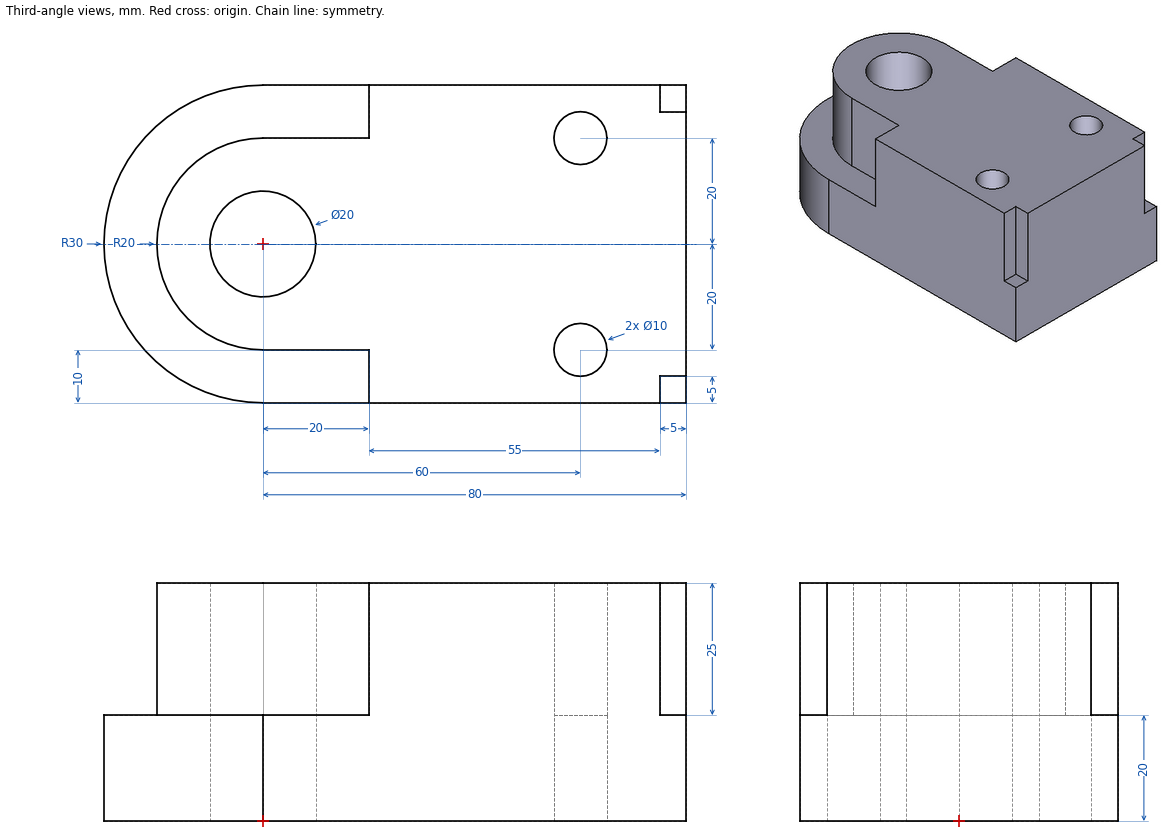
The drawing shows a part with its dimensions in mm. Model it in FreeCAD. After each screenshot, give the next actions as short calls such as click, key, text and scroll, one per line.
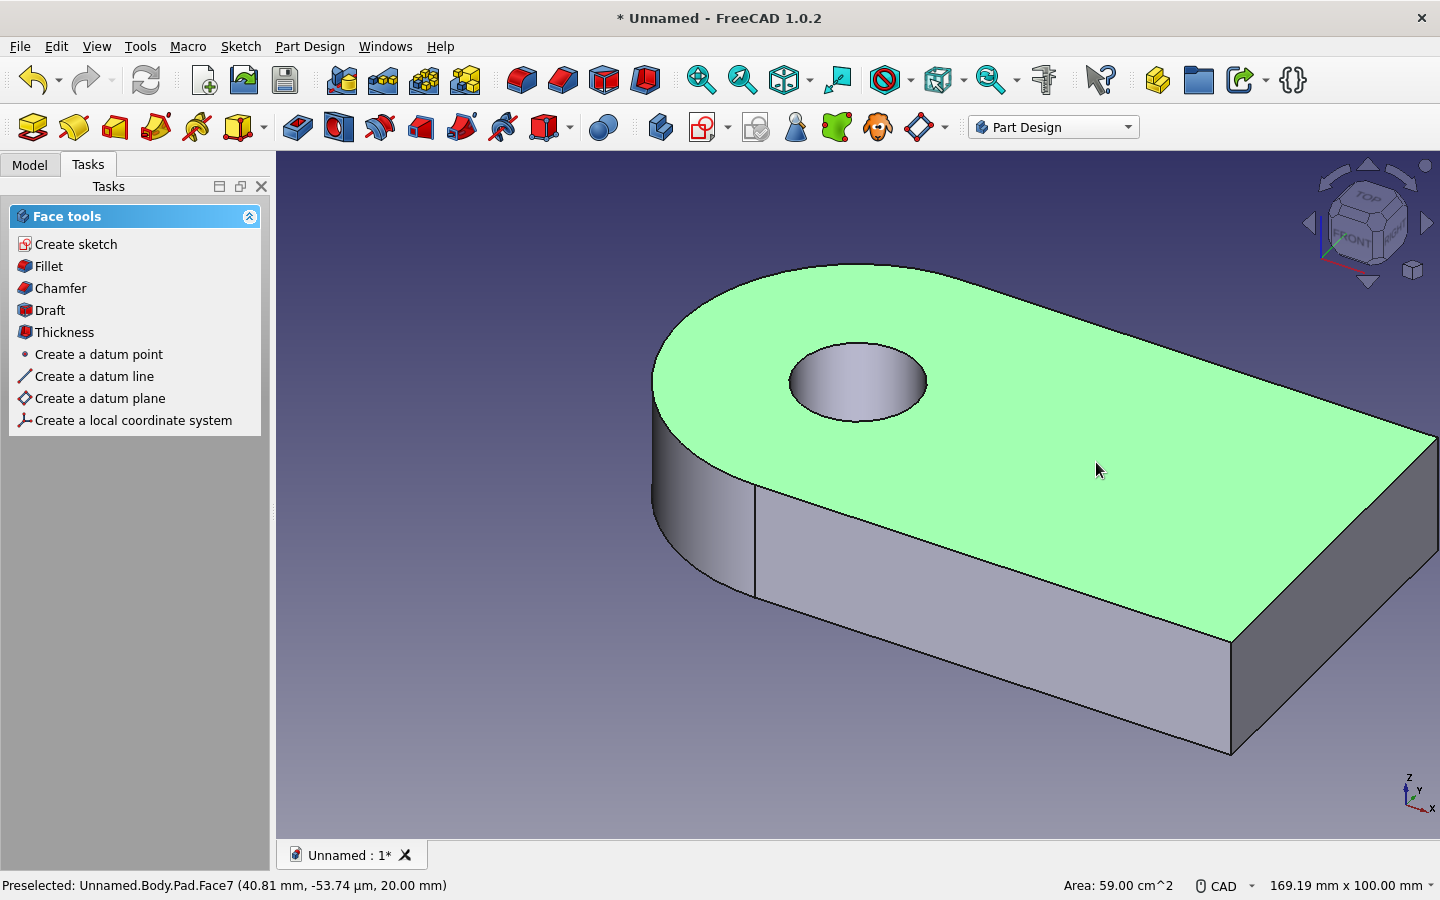
click(702, 128)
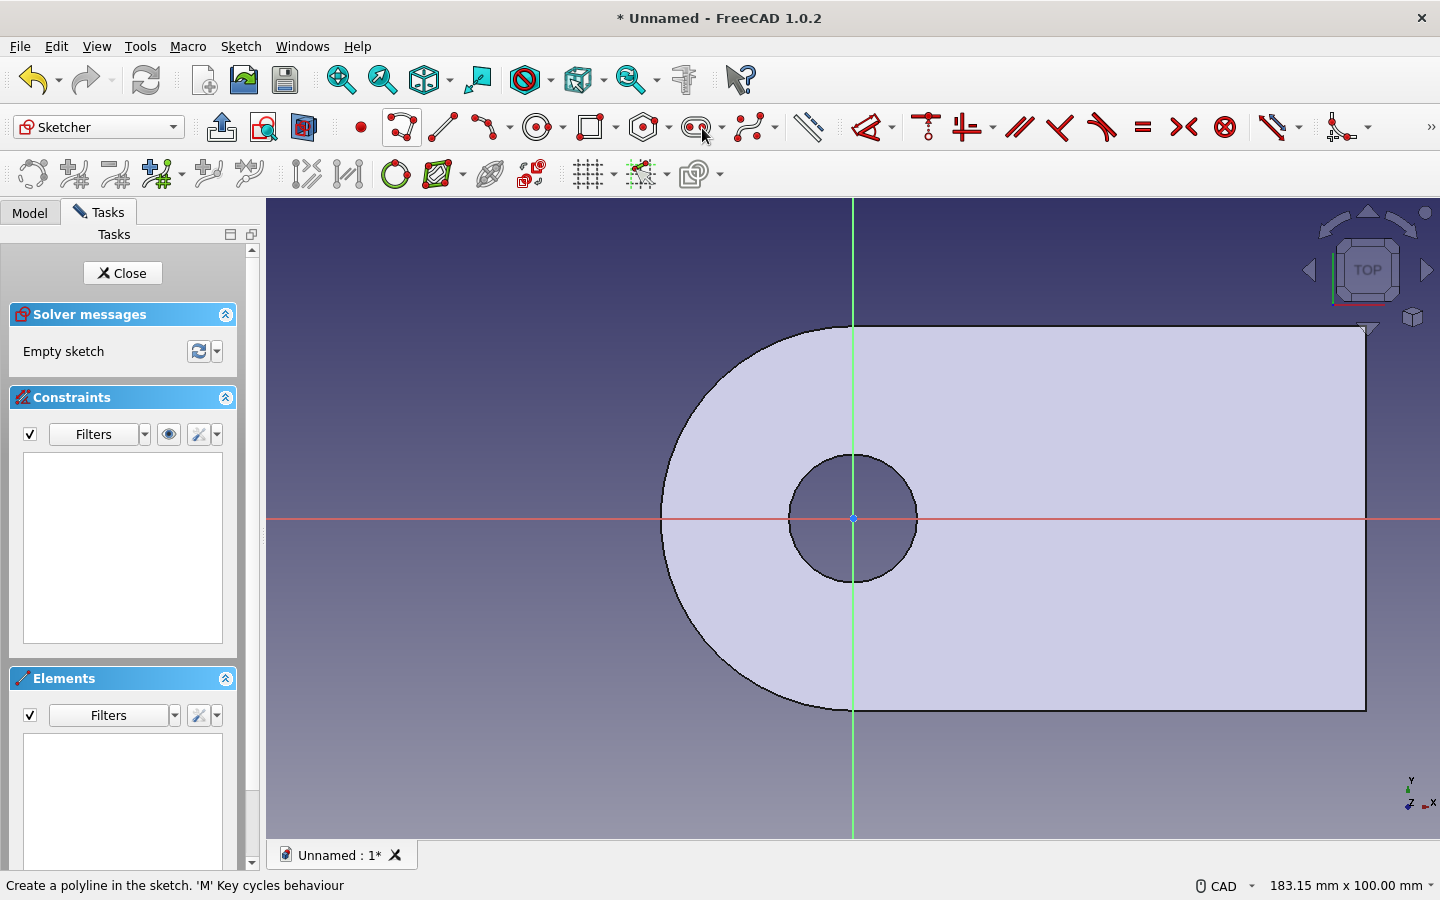
scroll(294, 519, down, 1)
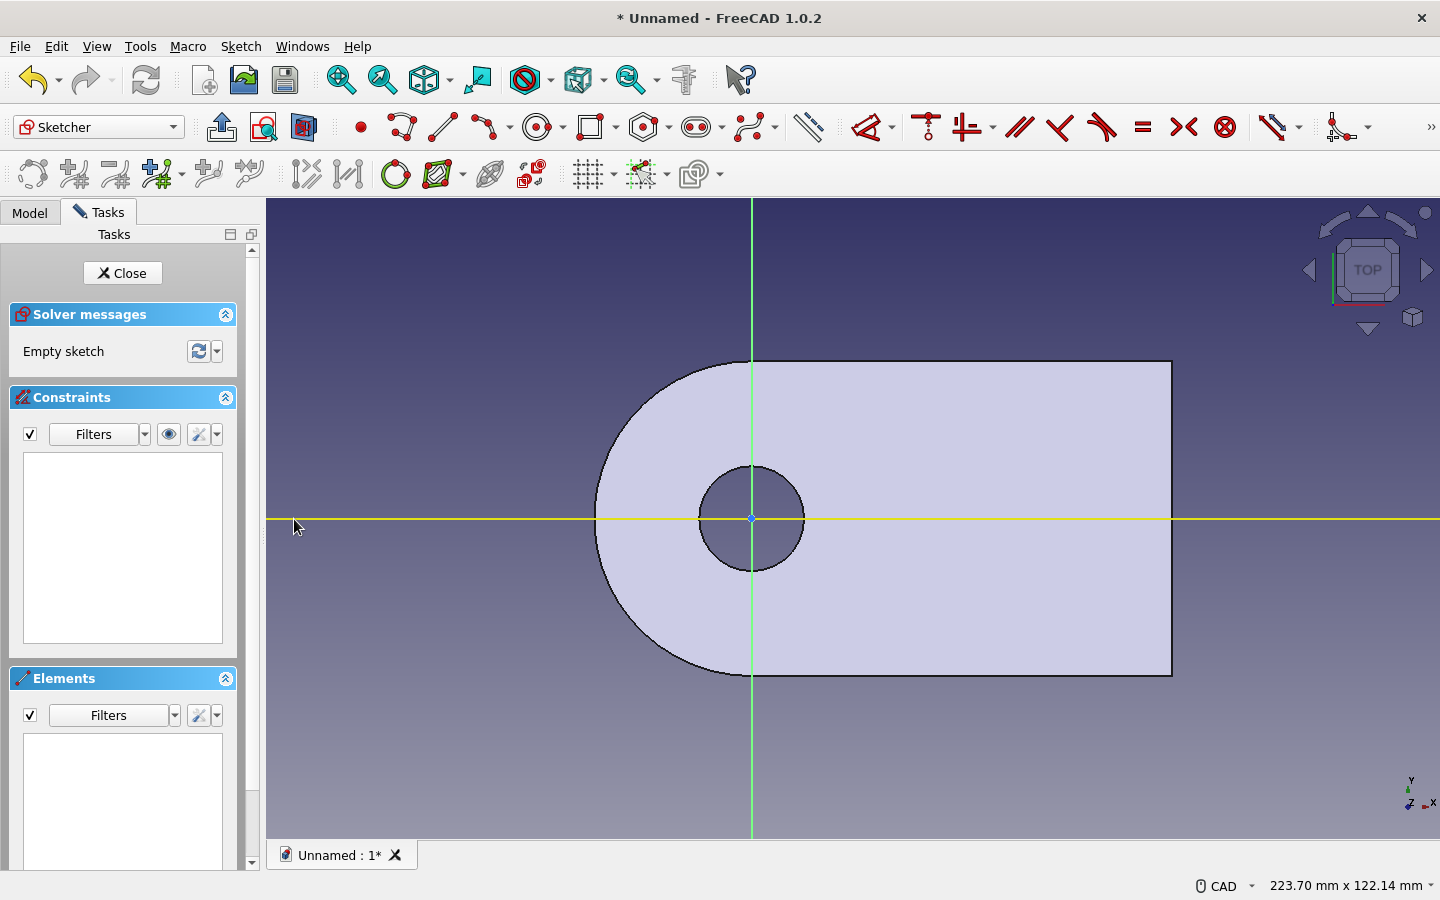
click(402, 128)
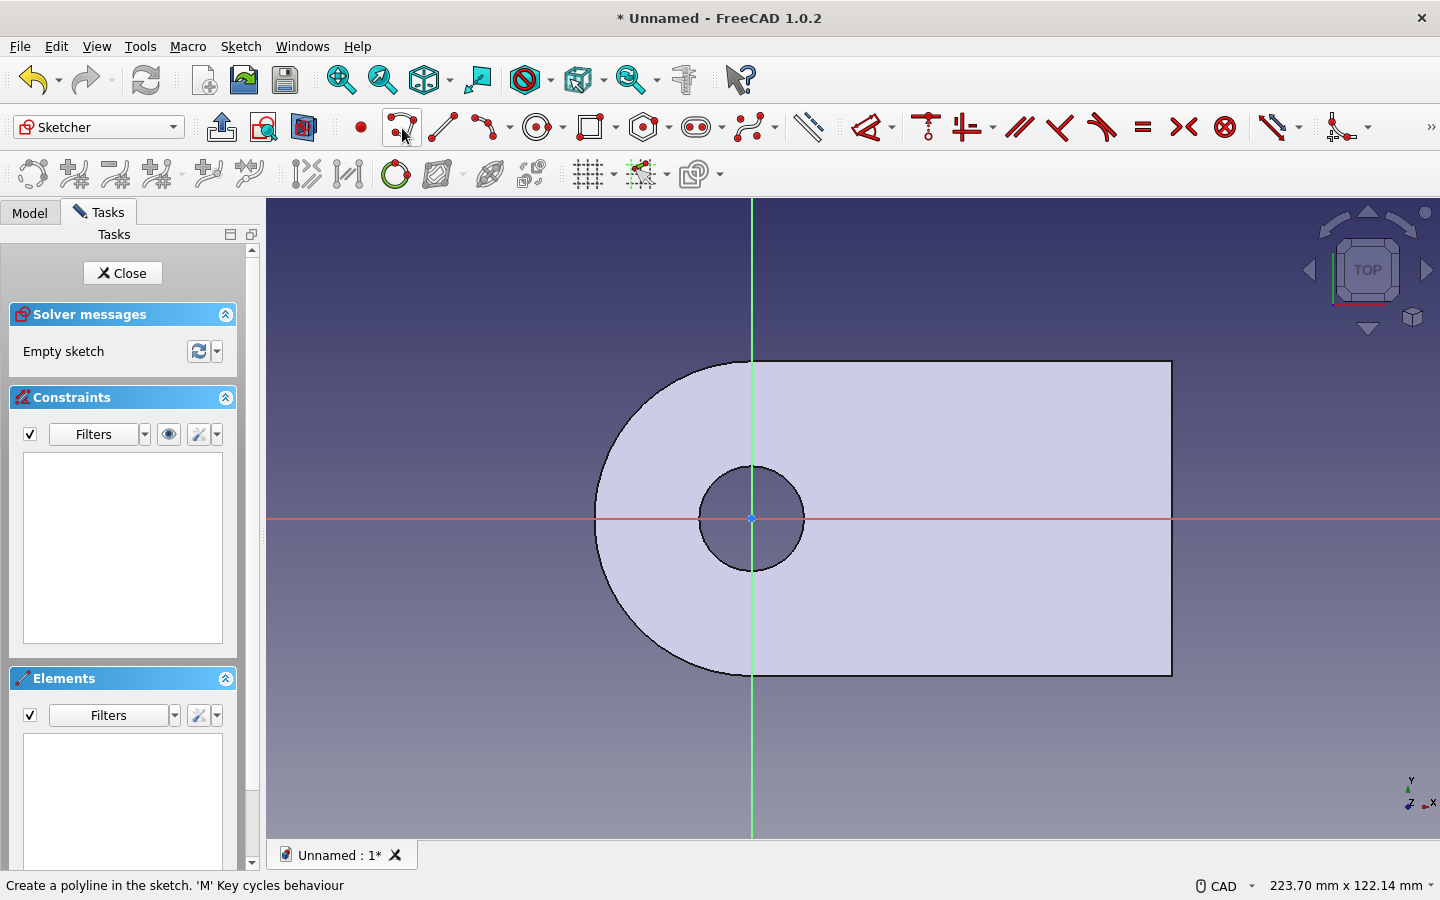
click(752, 624)
click(857, 624)
click(857, 676)
click(1145, 676)
click(1145, 650)
click(1172, 650)
click(1172, 387)
click(1145, 387)
click(1145, 361)
click(857, 361)
click(857, 414)
click(752, 414)
right_click(752, 414)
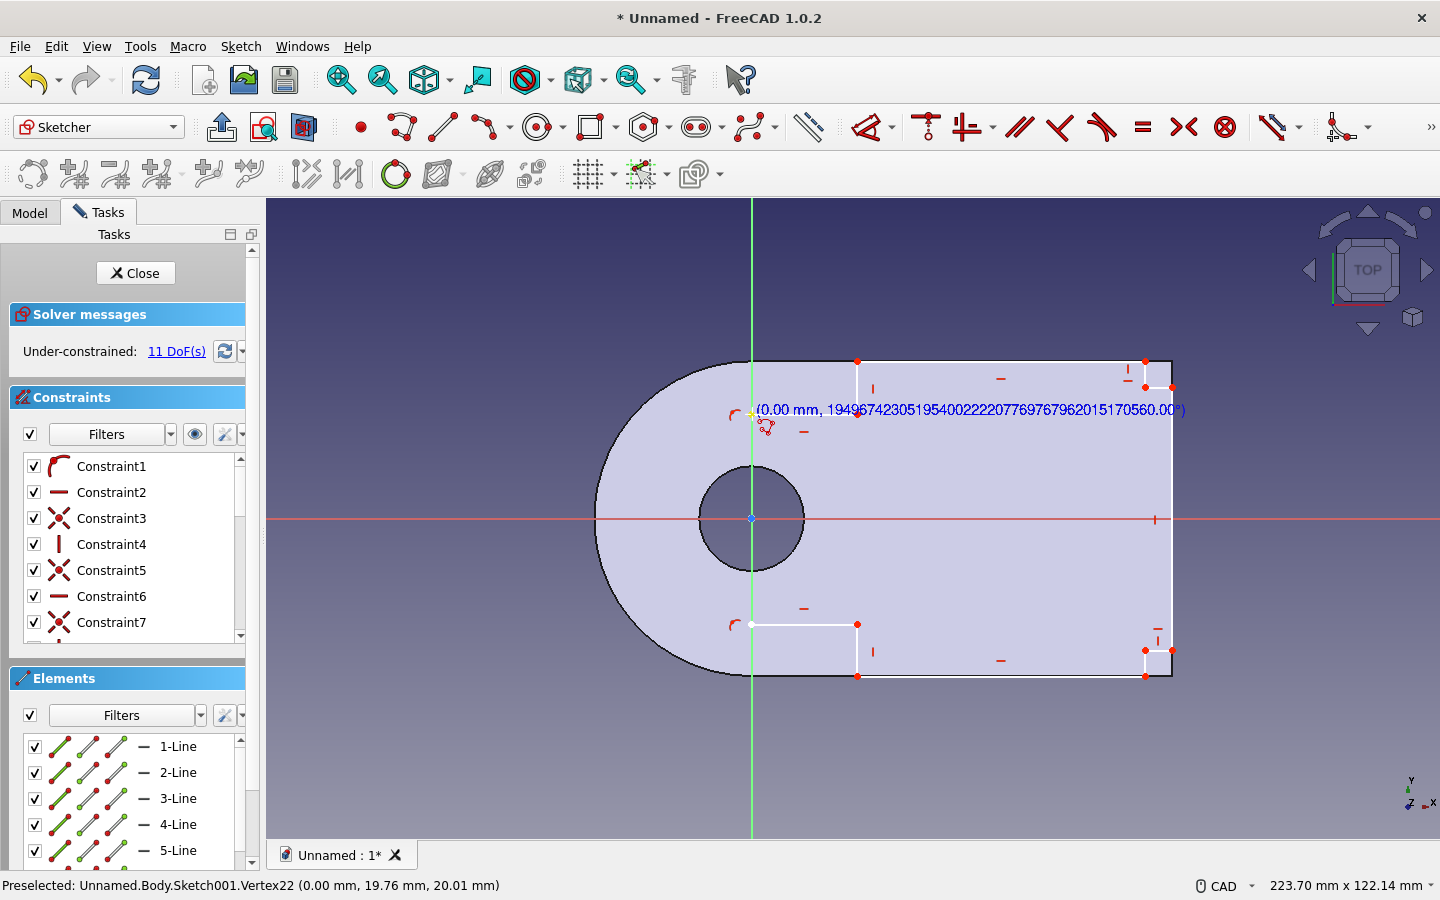
key(g)
key(3)
key(a)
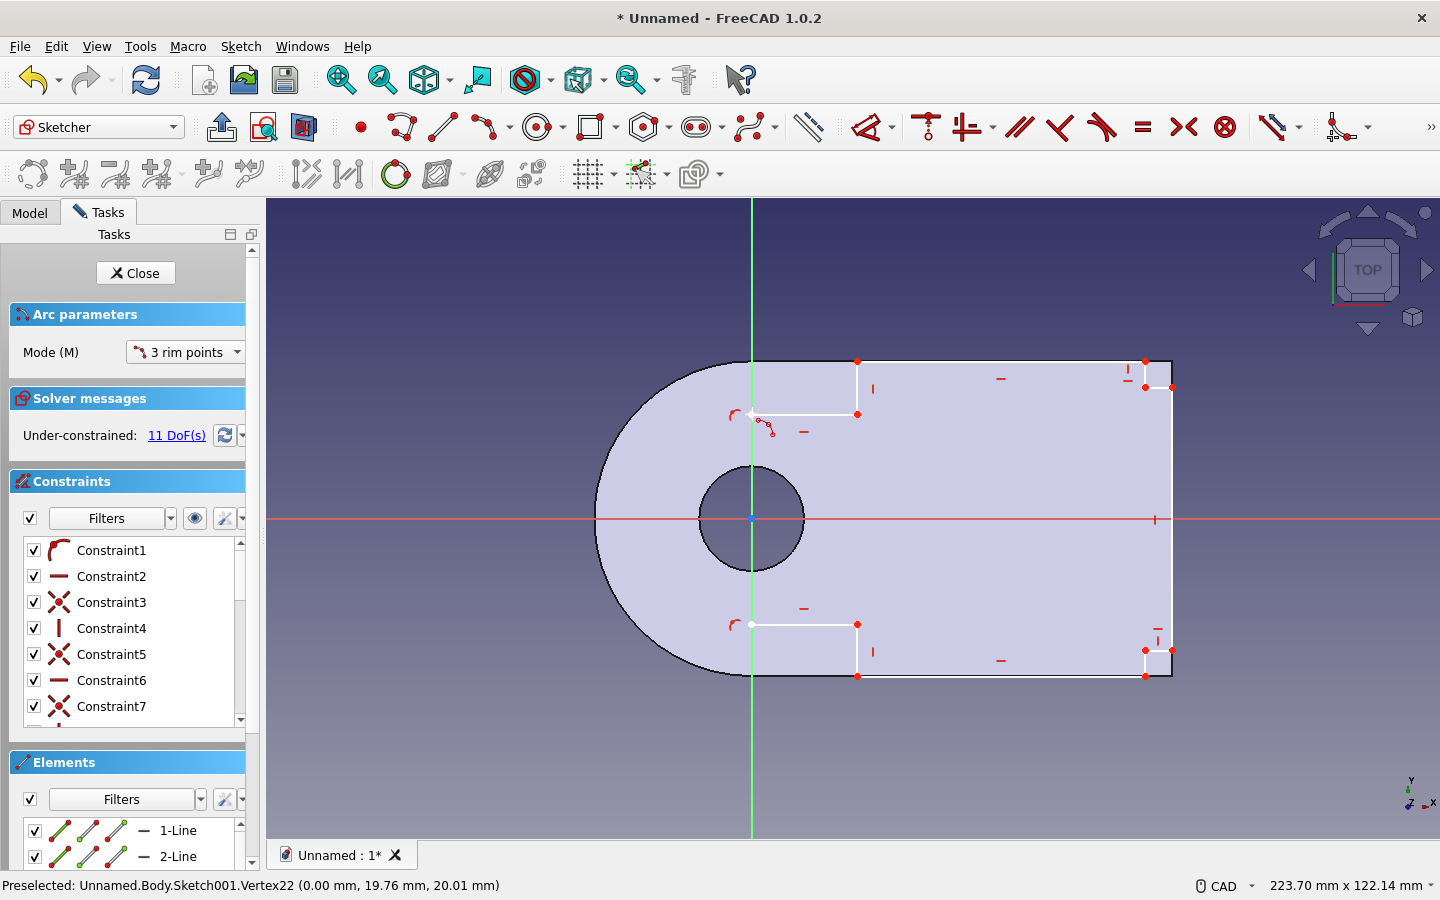
click(752, 415)
click(752, 625)
click(652, 486)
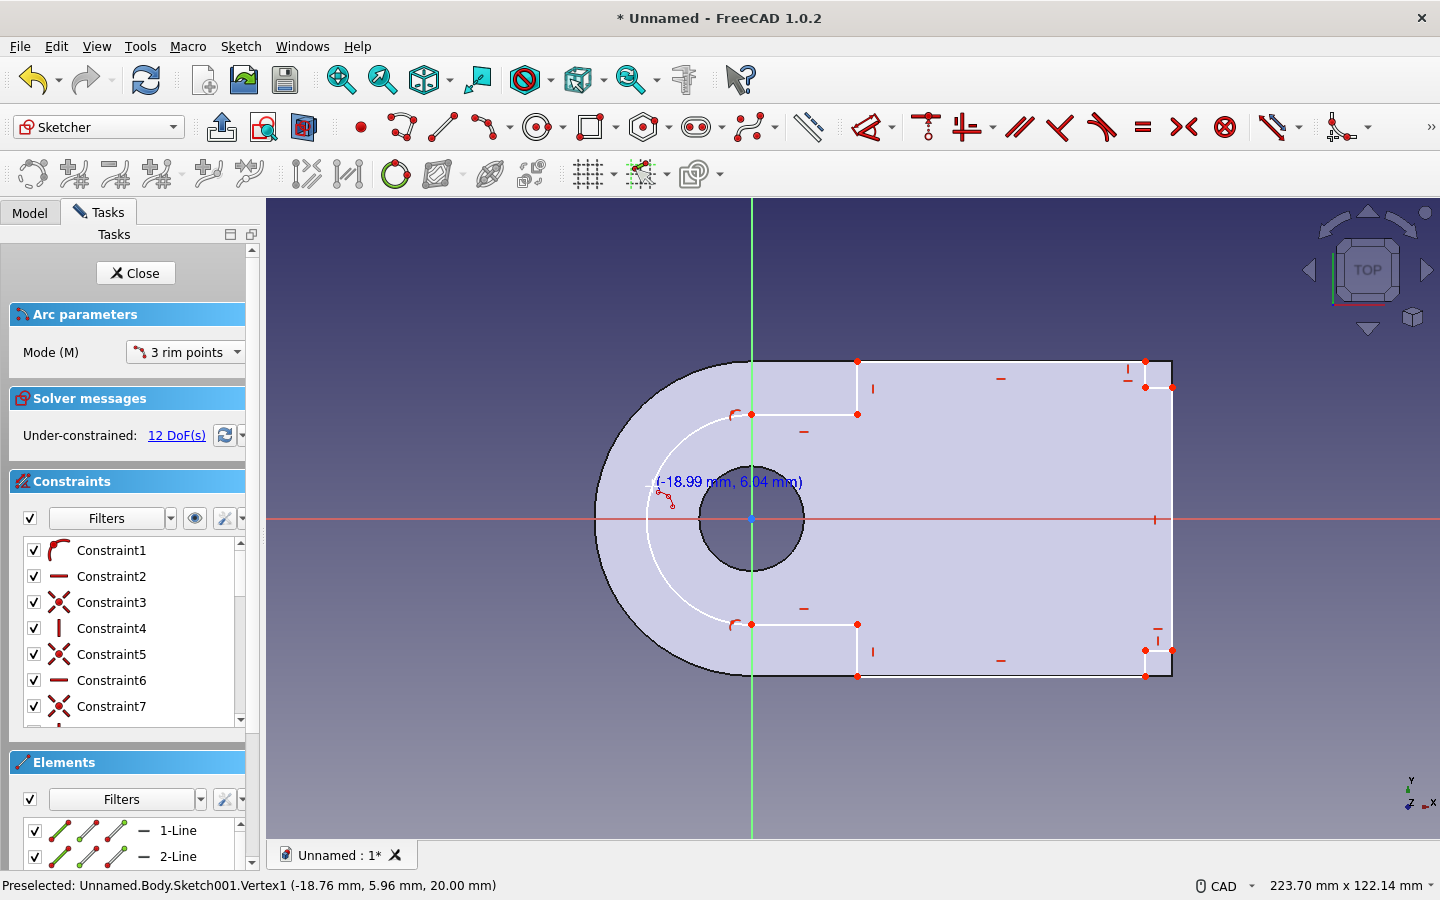
click(536, 128)